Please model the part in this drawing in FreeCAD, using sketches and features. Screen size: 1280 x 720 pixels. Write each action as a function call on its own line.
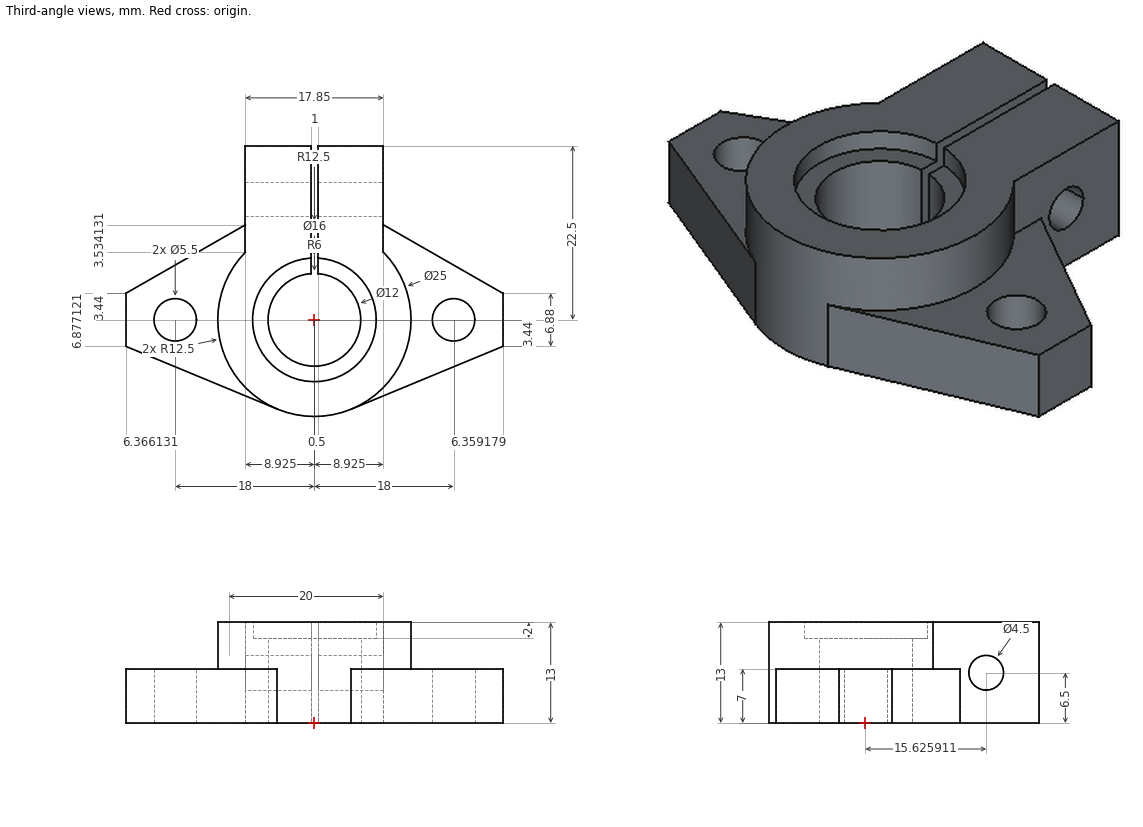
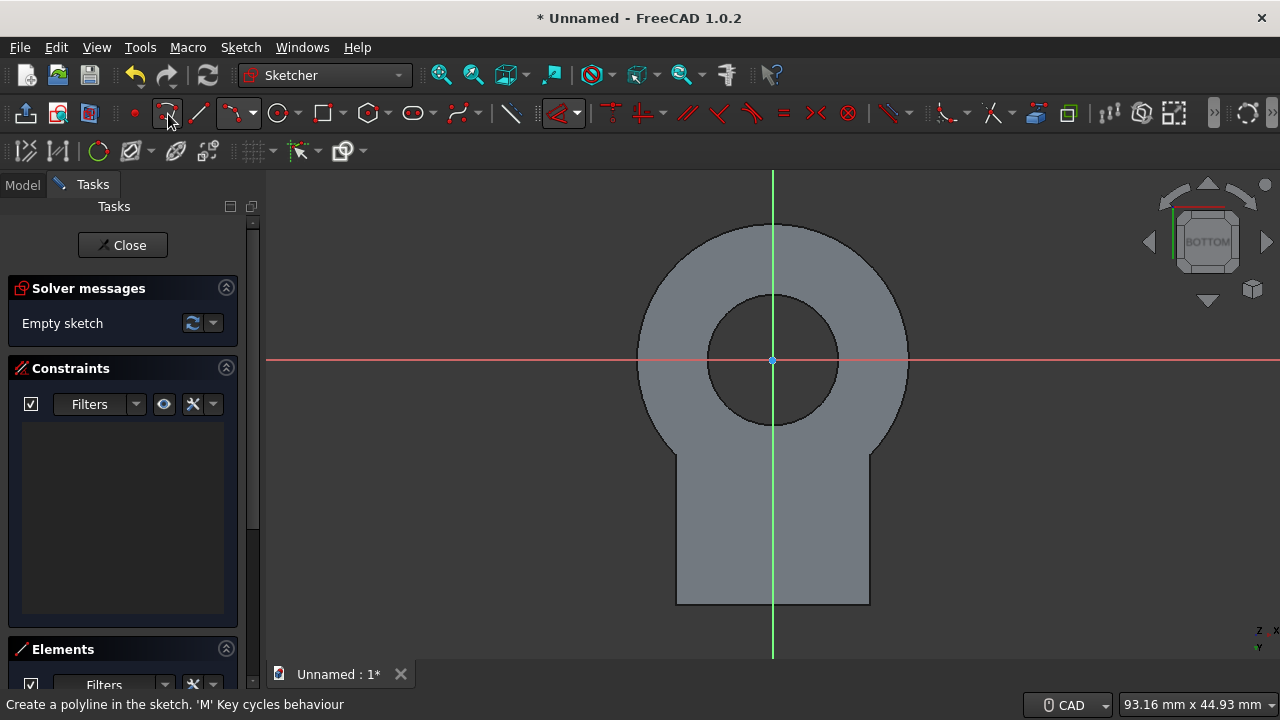
click(676, 455)
click(676, 494)
click(508, 398)
click(508, 323)
click(721, 234)
right_click(721, 234)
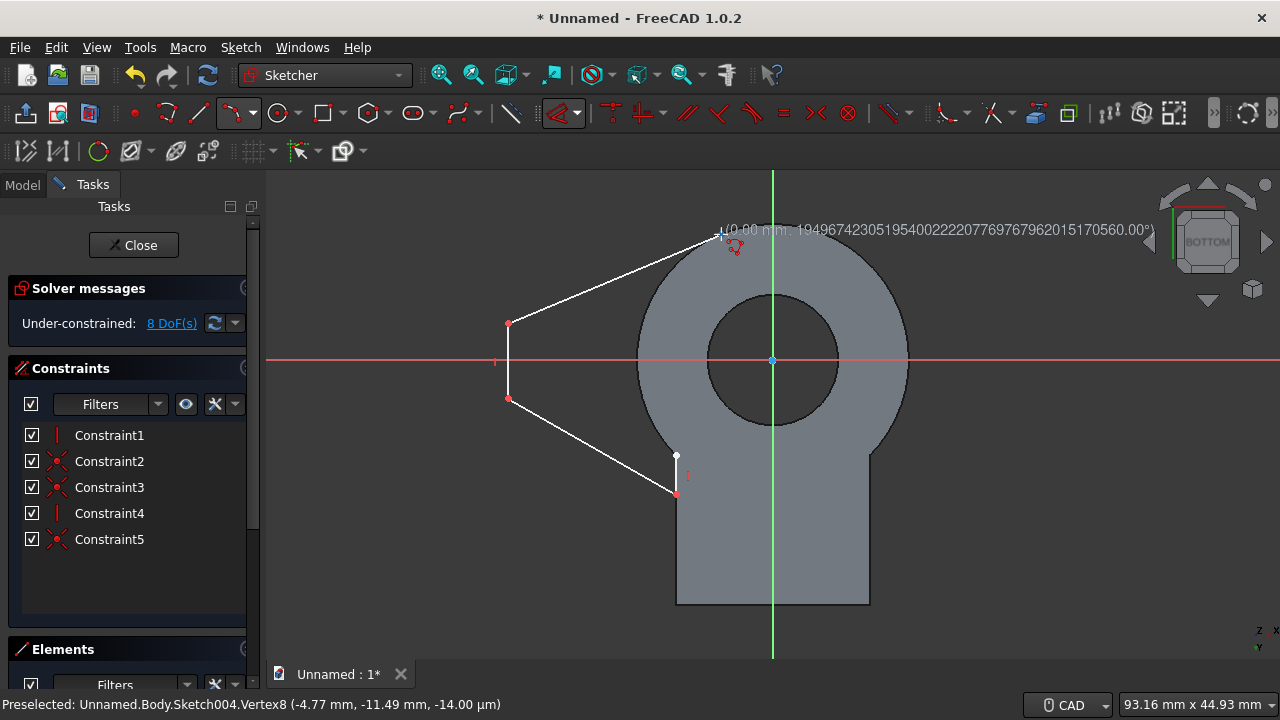
click(232, 114)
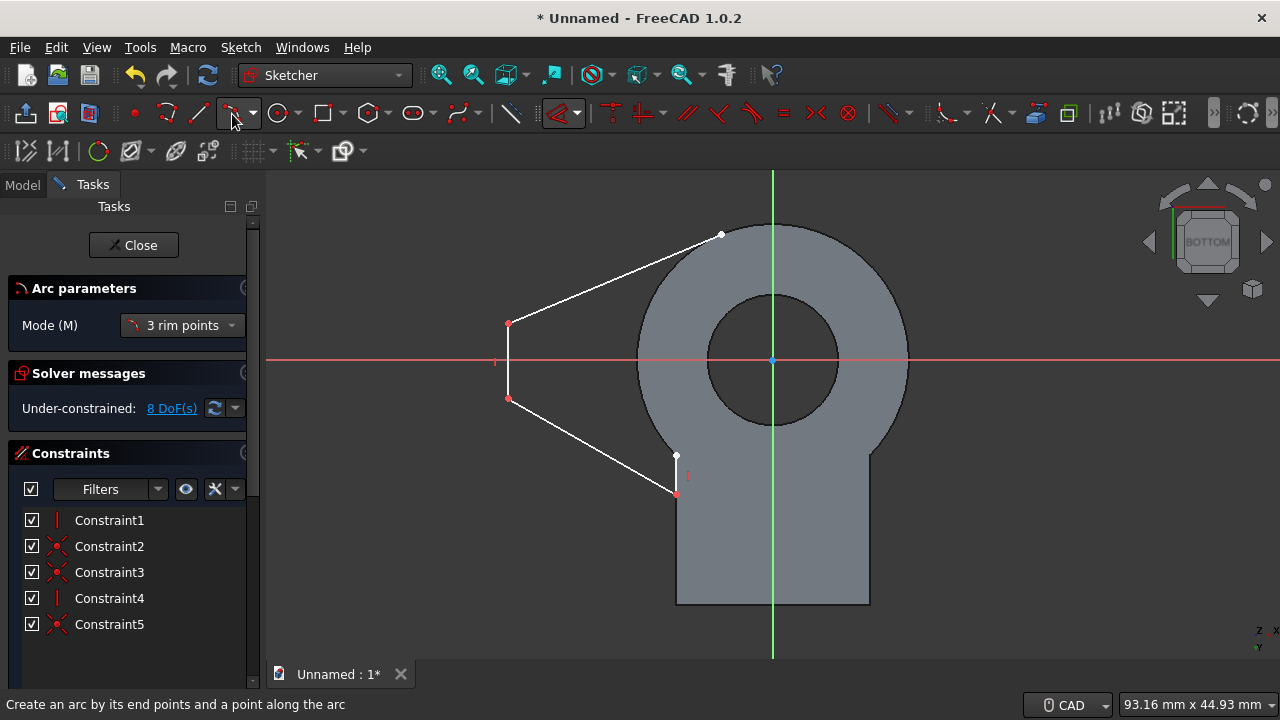
click(721, 235)
click(676, 456)
click(640, 333)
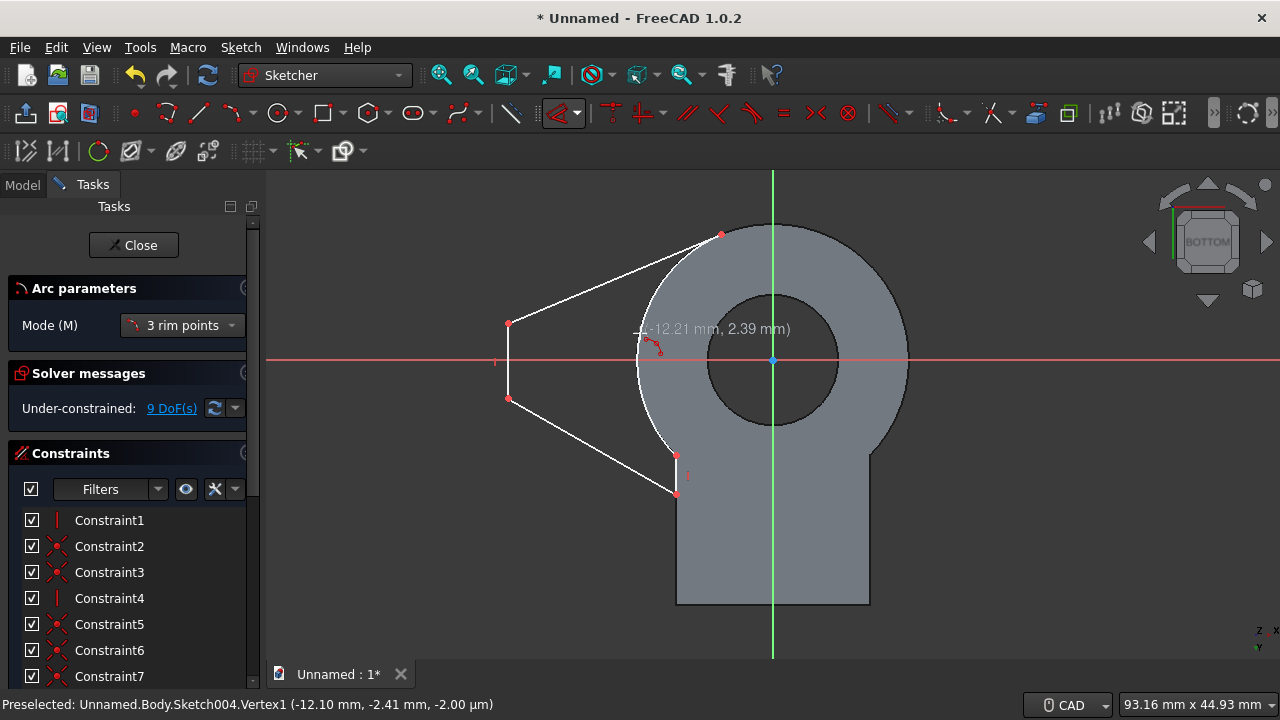
click(168, 114)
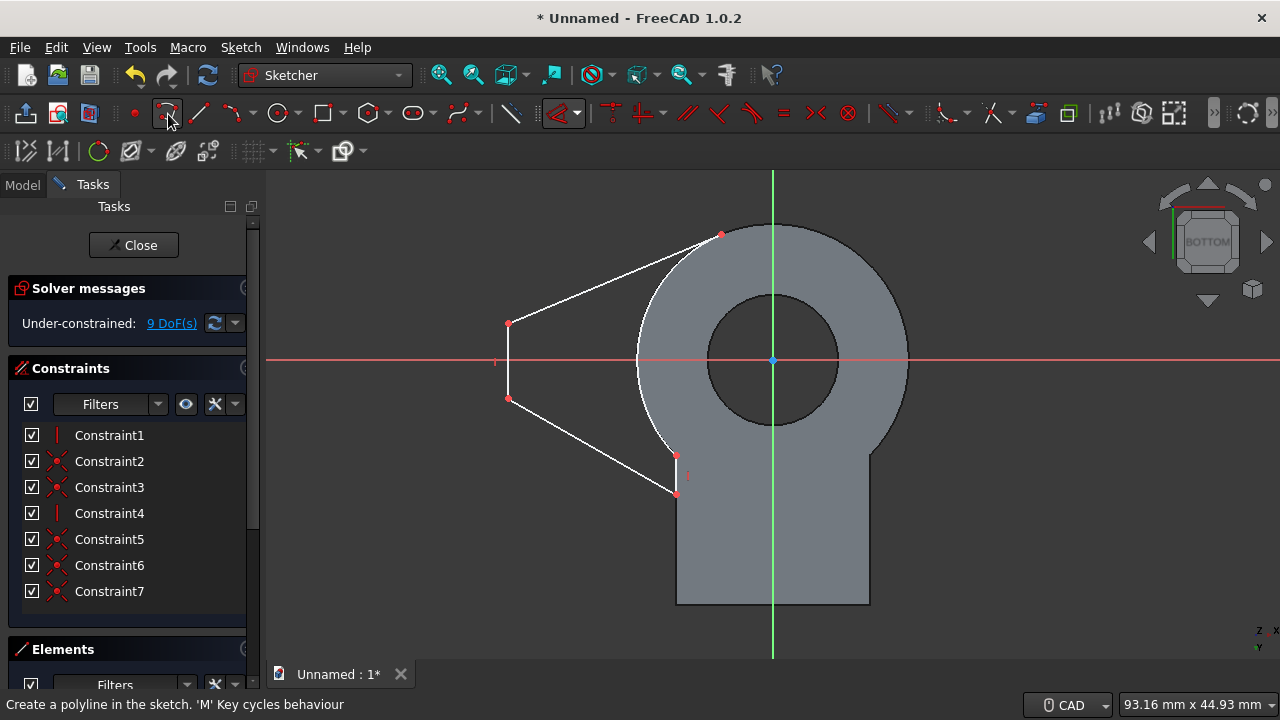
click(825, 234)
click(1038, 323)
click(1038, 398)
click(870, 494)
click(870, 455)
right_click(870, 455)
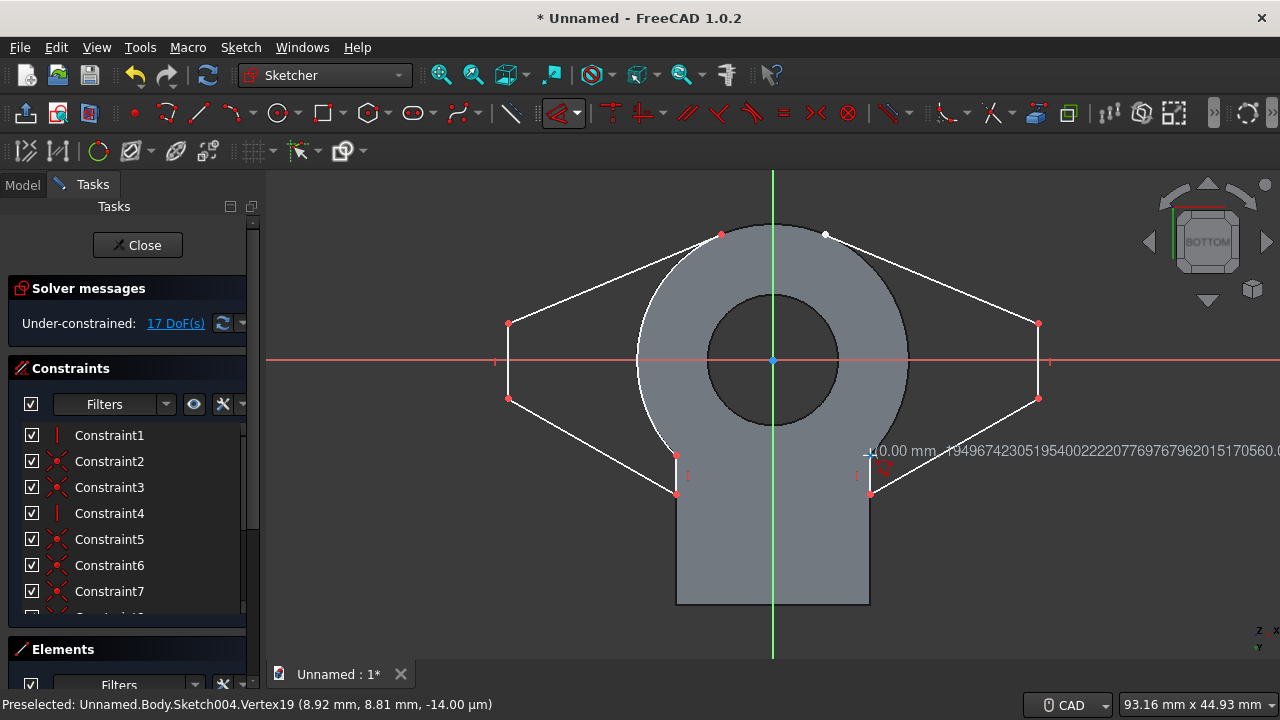
click(232, 114)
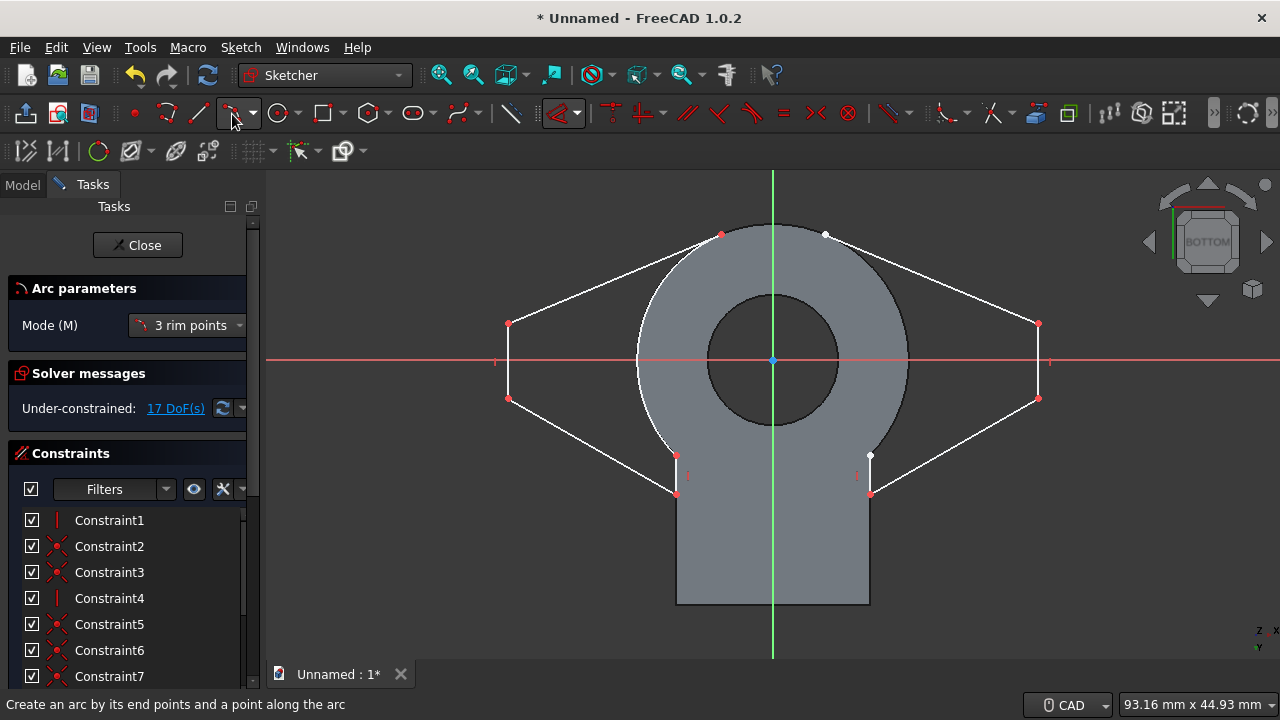
click(870, 456)
click(825, 235)
click(906, 333)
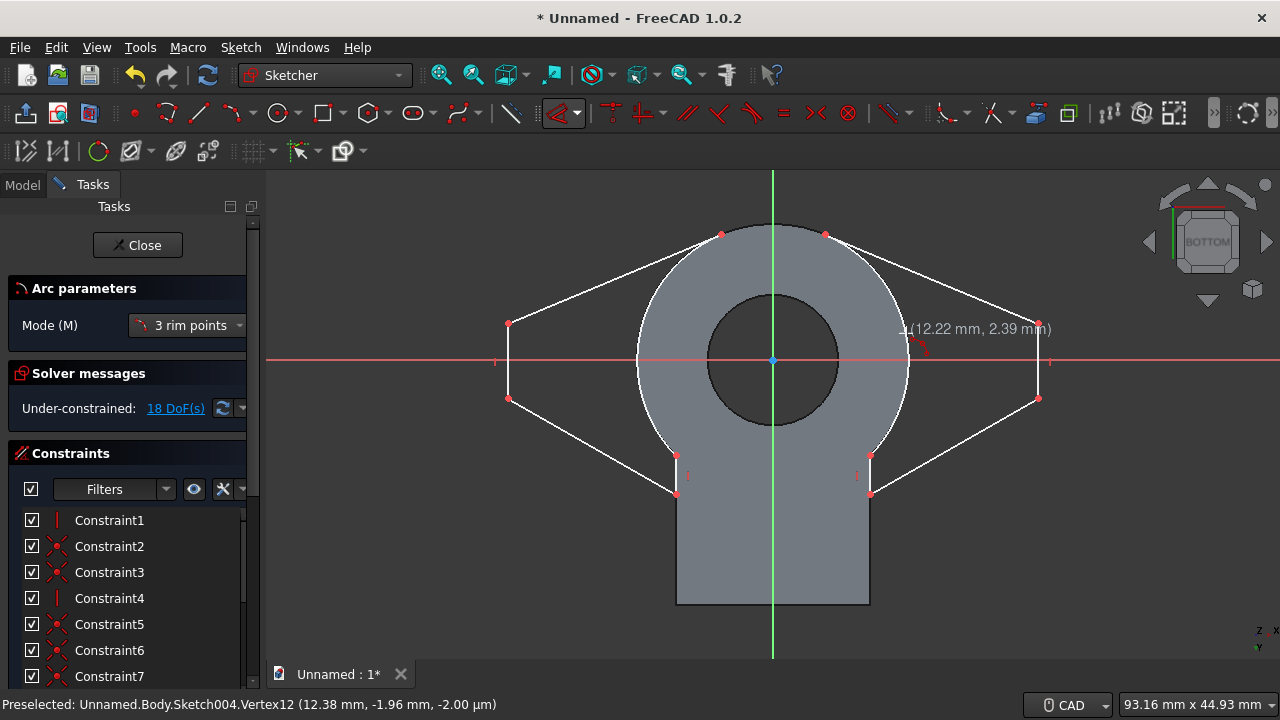
click(278, 114)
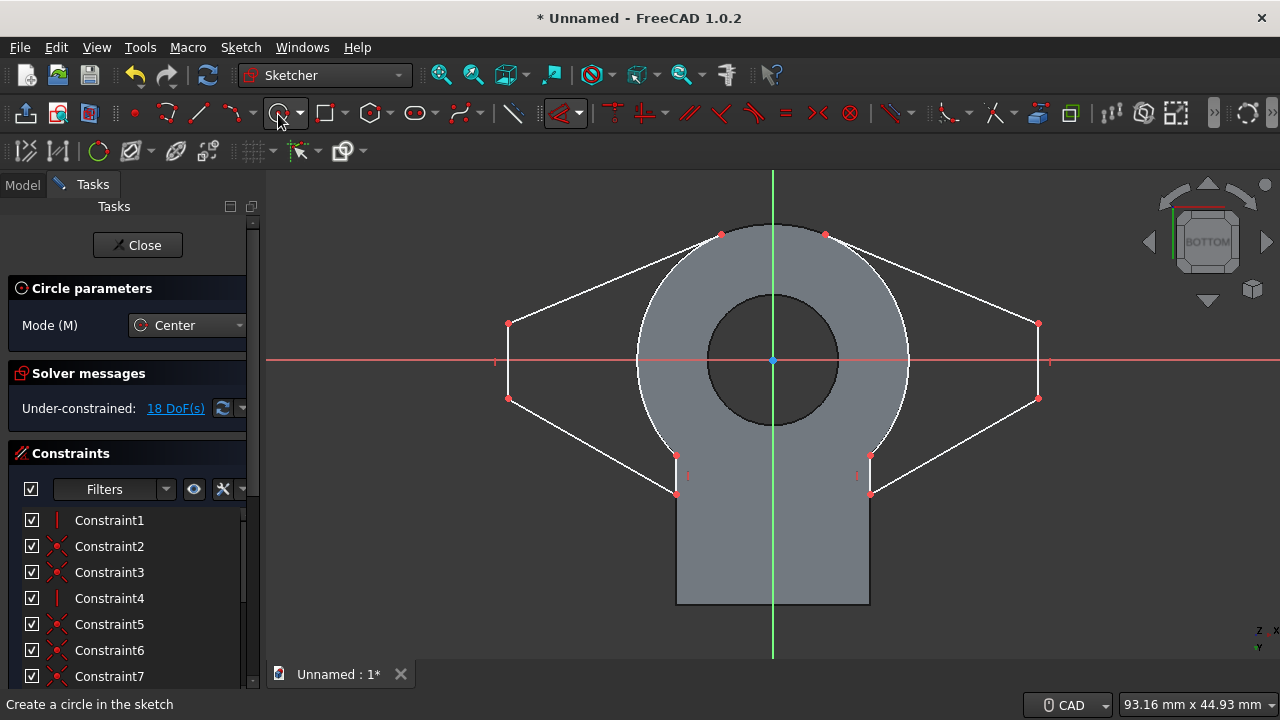
click(577, 360)
click(598, 339)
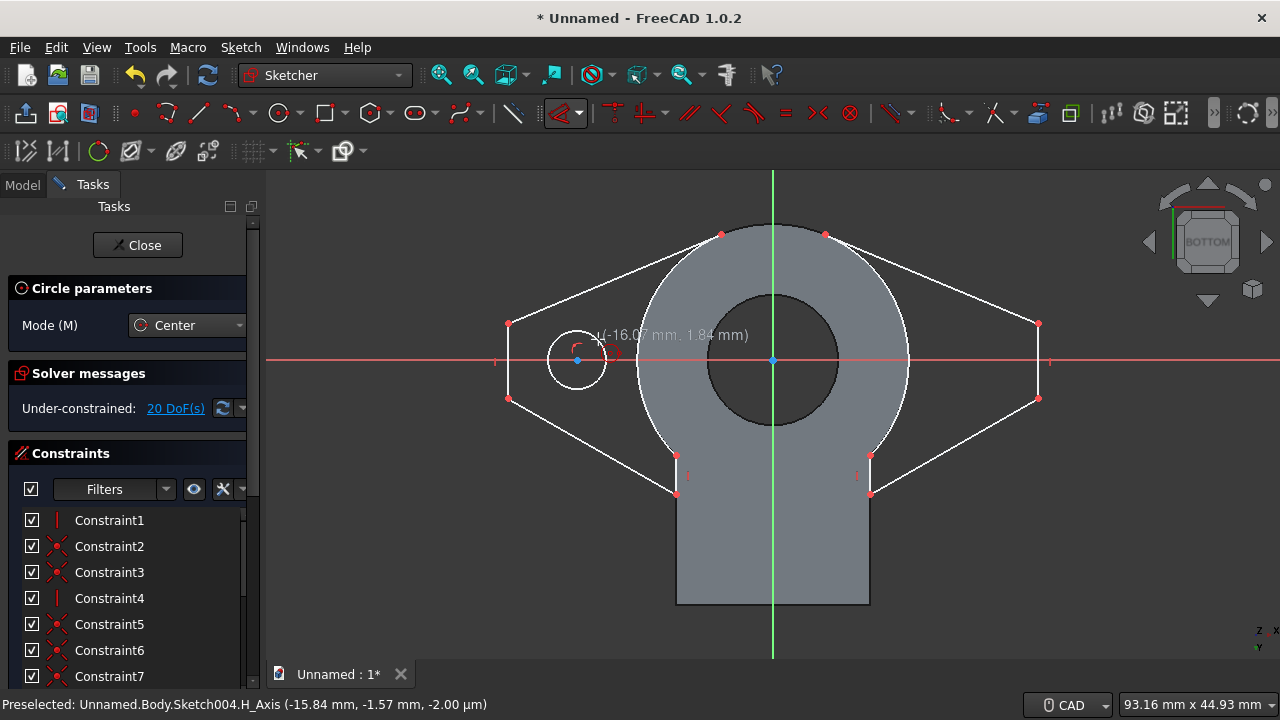
click(969, 360)
click(990, 339)
key(Escape)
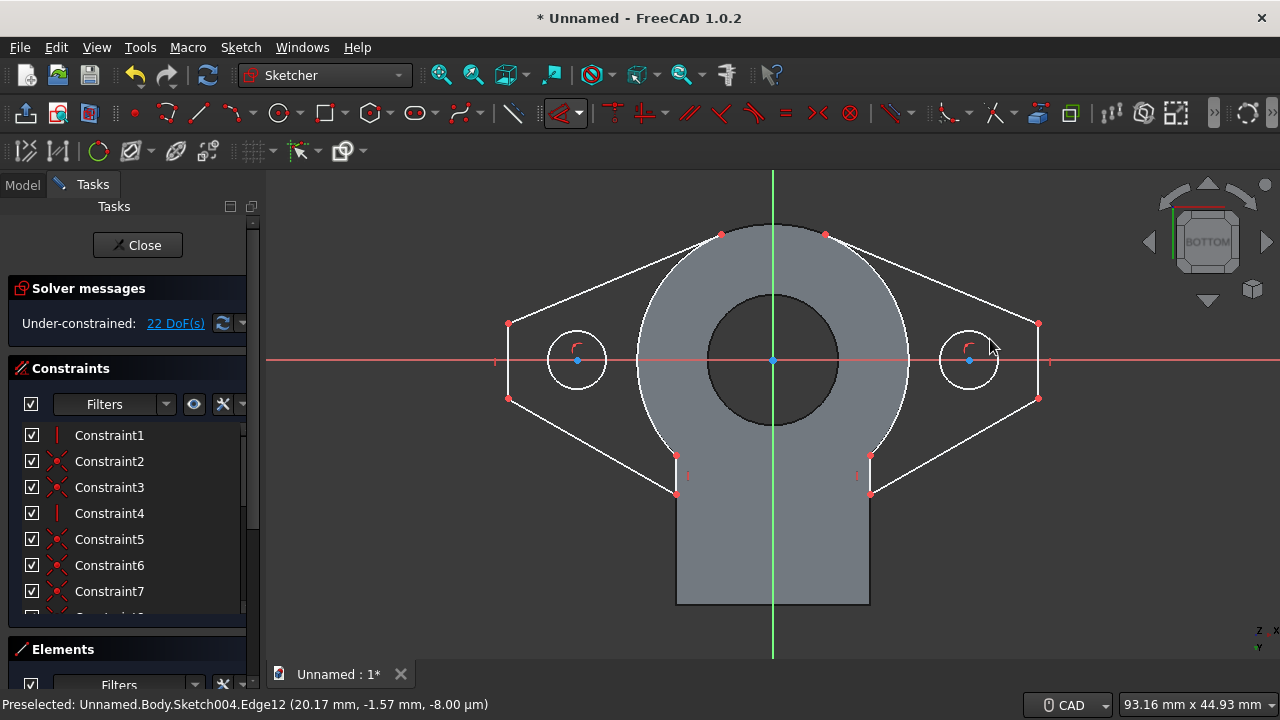
click(572, 297)